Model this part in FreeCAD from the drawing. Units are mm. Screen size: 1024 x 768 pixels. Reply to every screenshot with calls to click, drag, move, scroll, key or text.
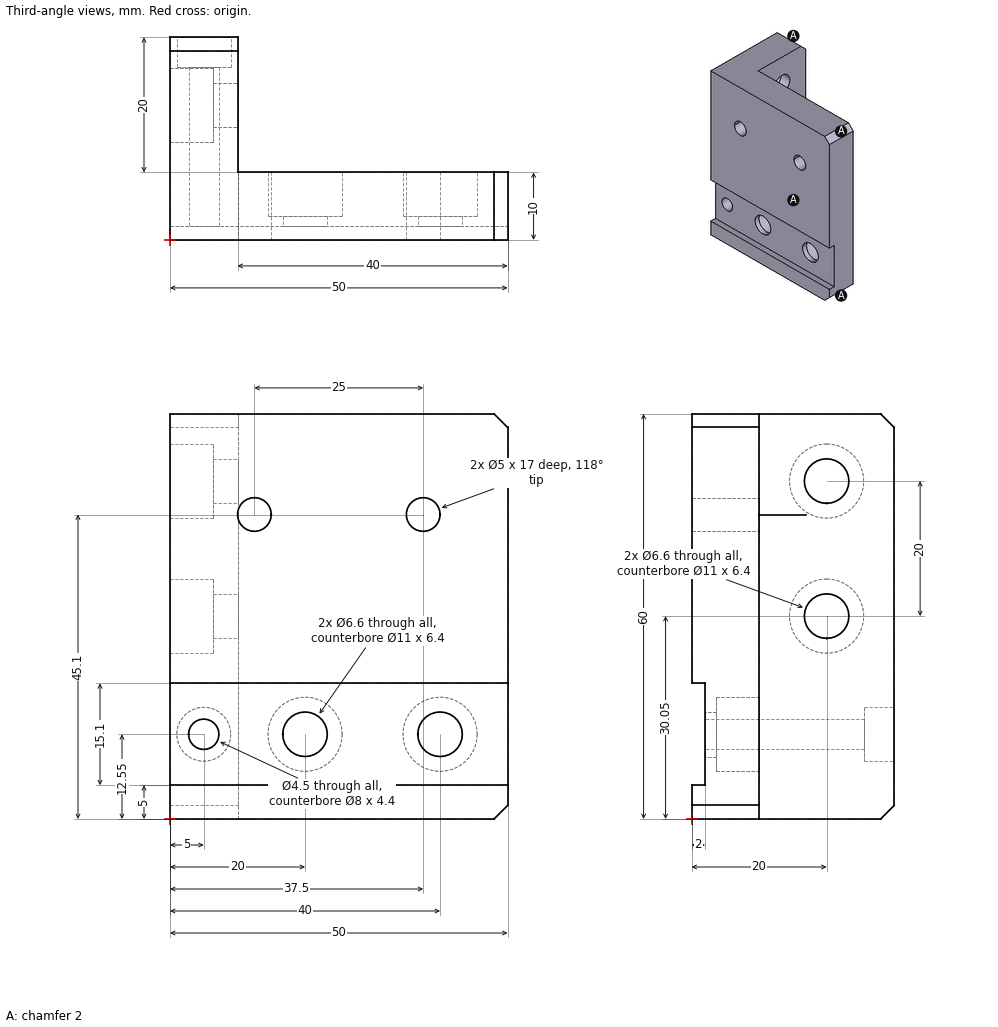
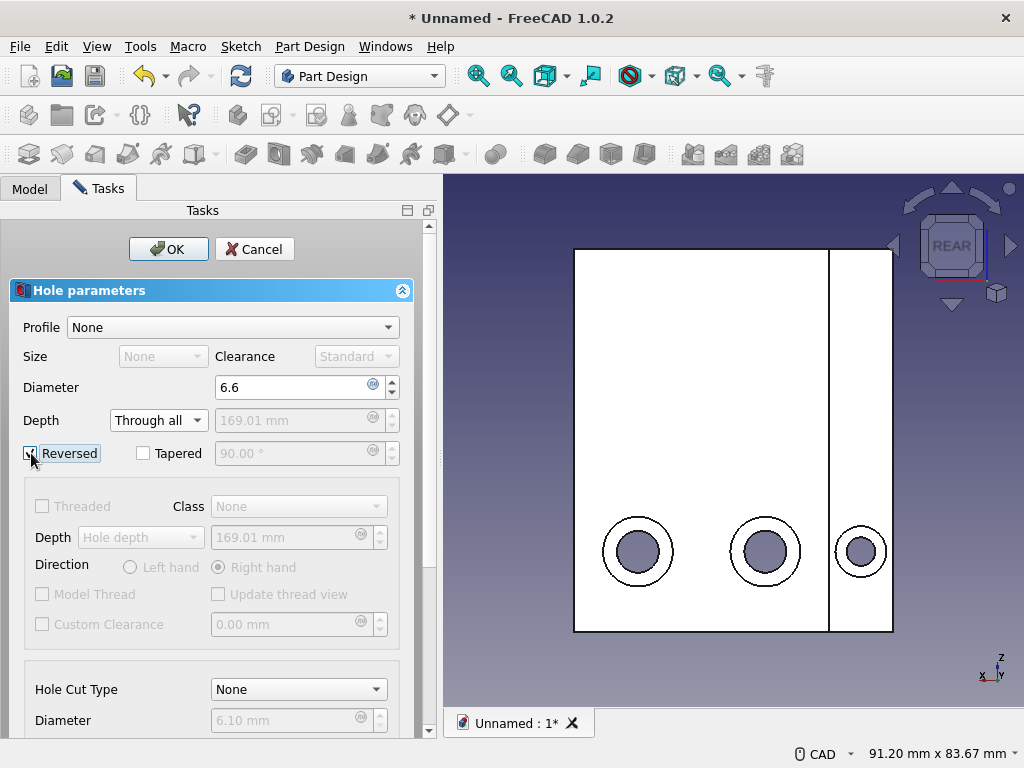
click(300, 690)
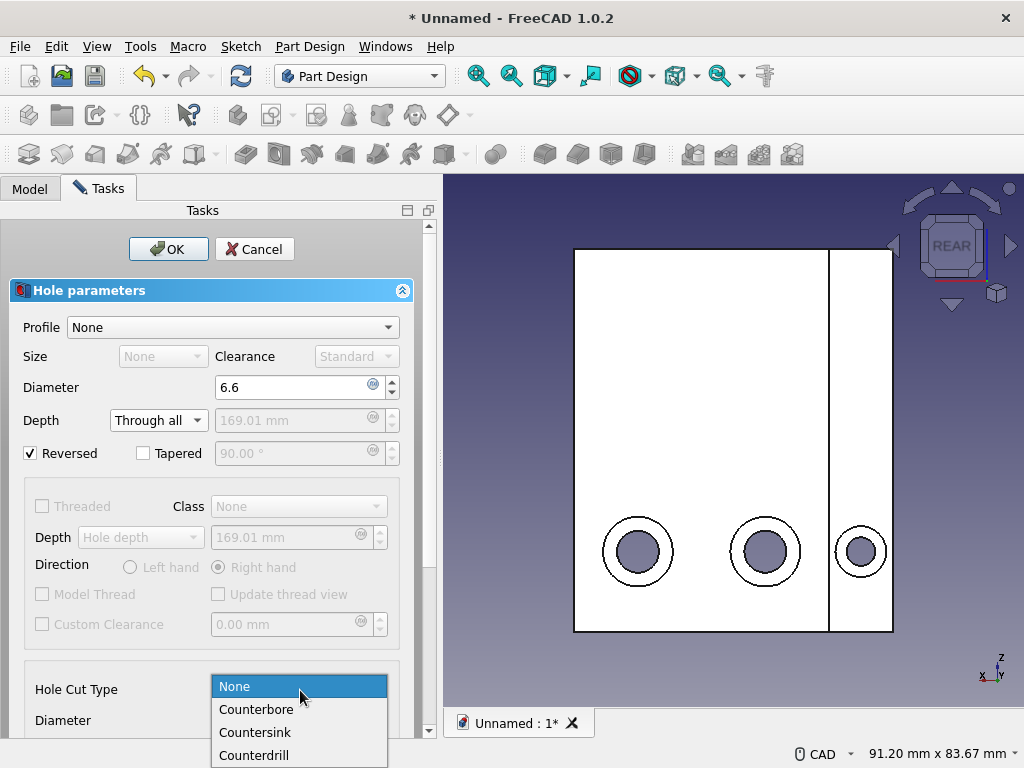
click(298, 710)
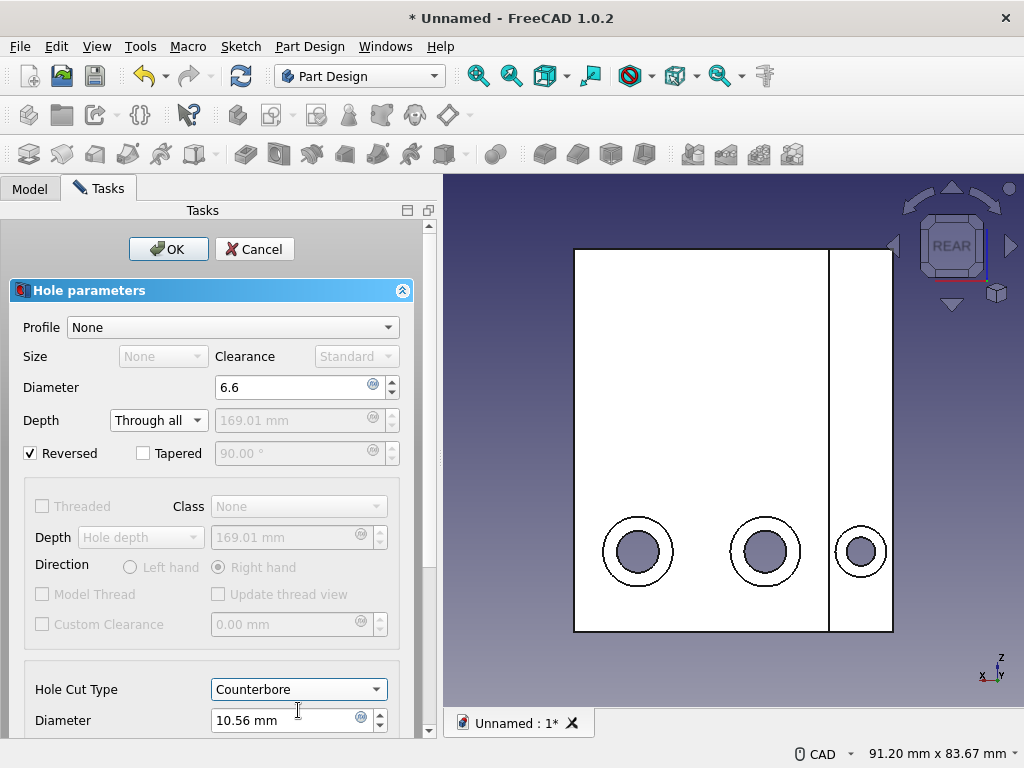
triple_click(292, 720)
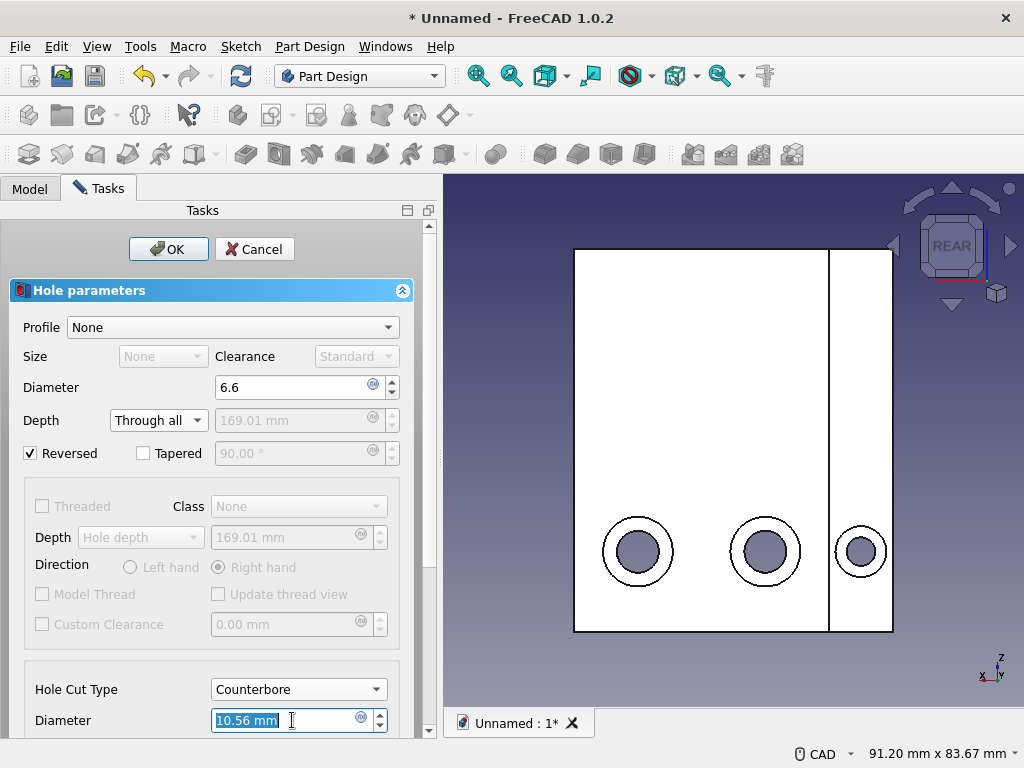
text(11)
key(Tab)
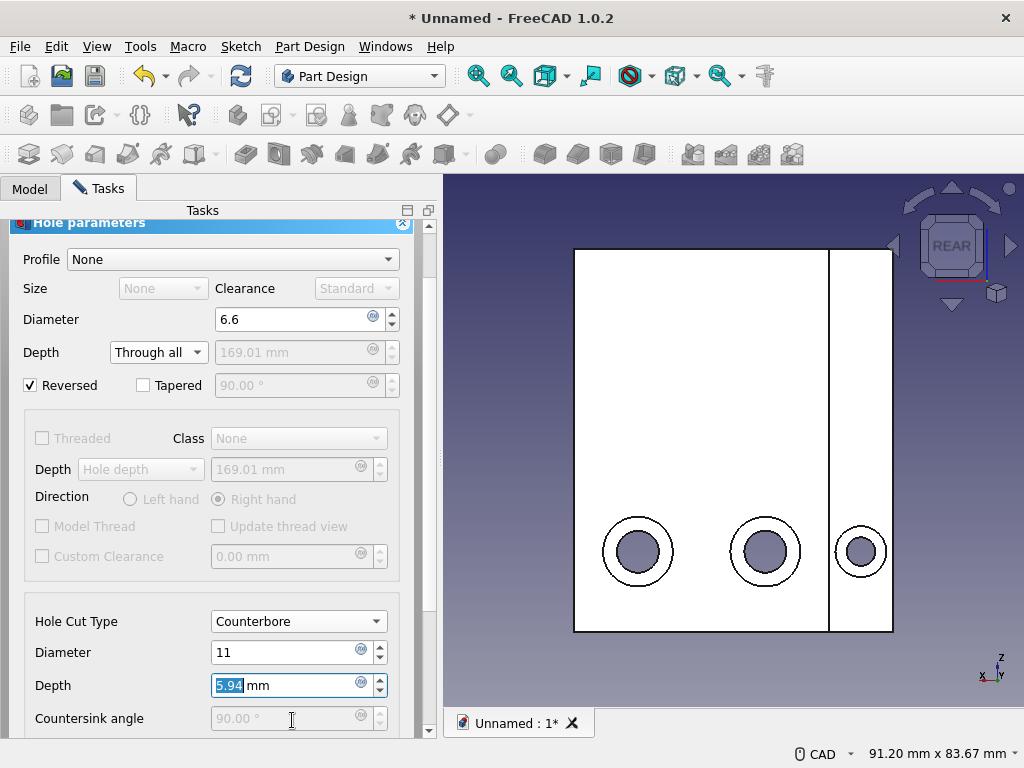
text(6.4)
key(Tab)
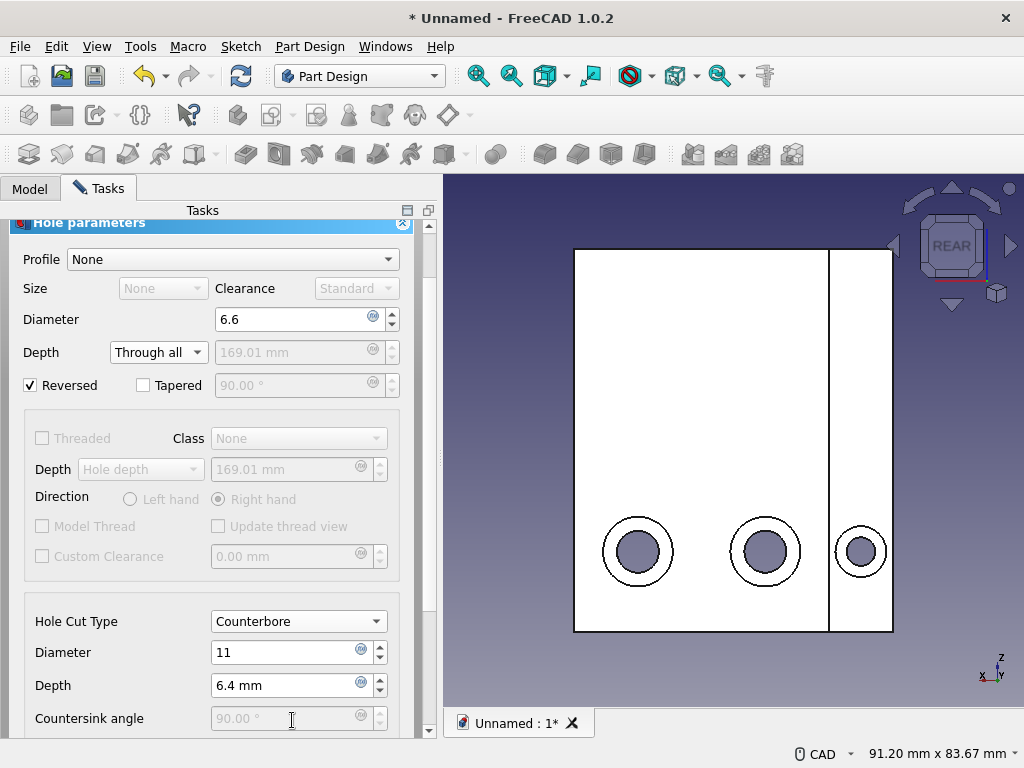
scroll(429, 479, up, 2)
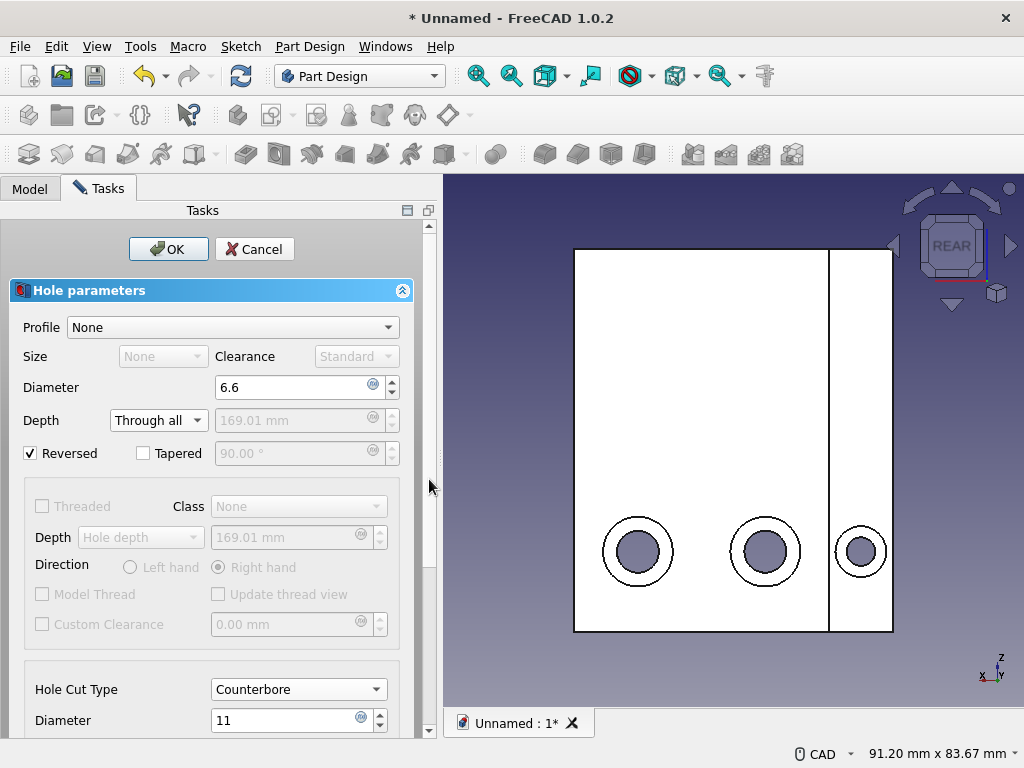
click(169, 249)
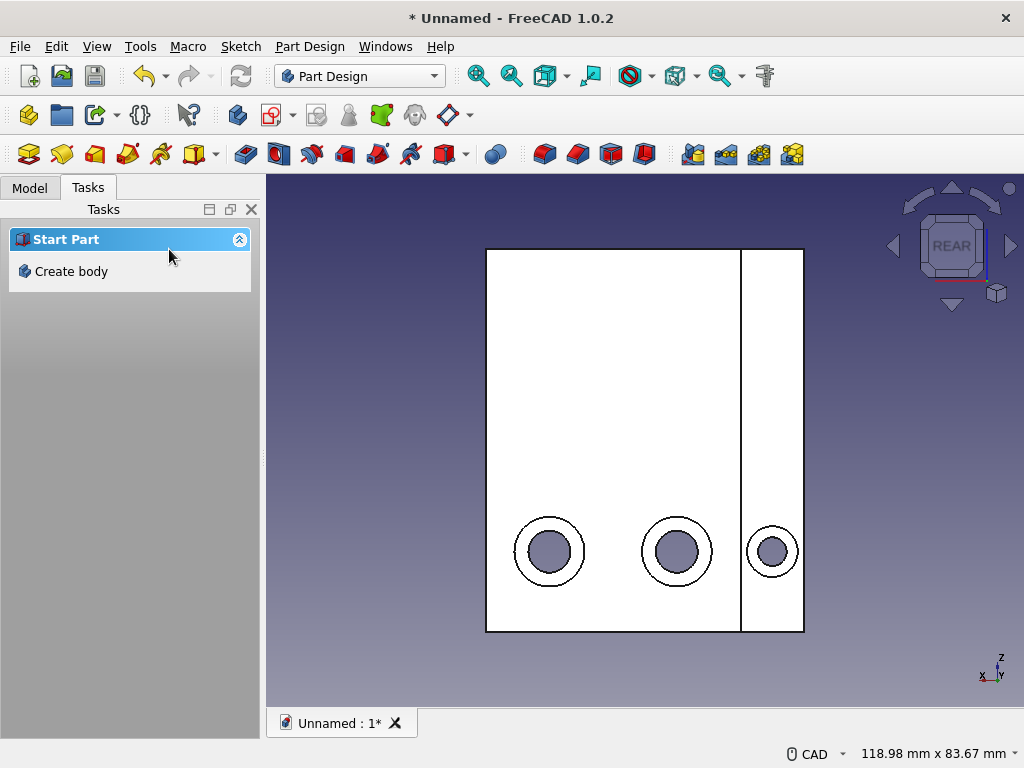
click(772, 248)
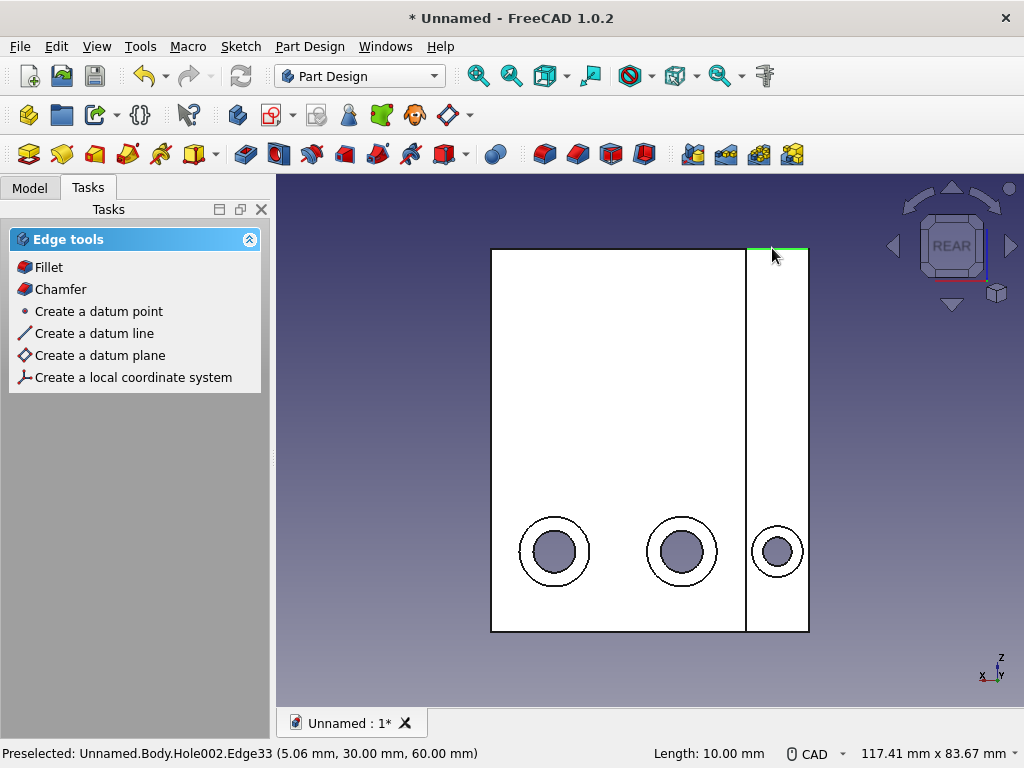
click(777, 631, ctrl)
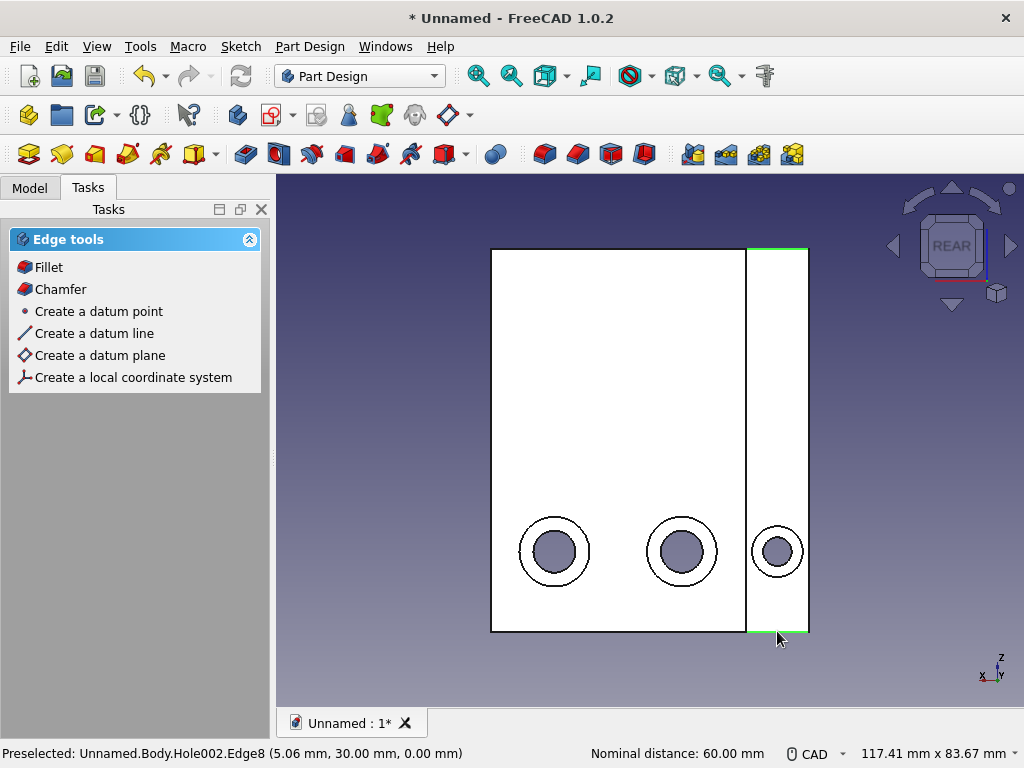
key(0)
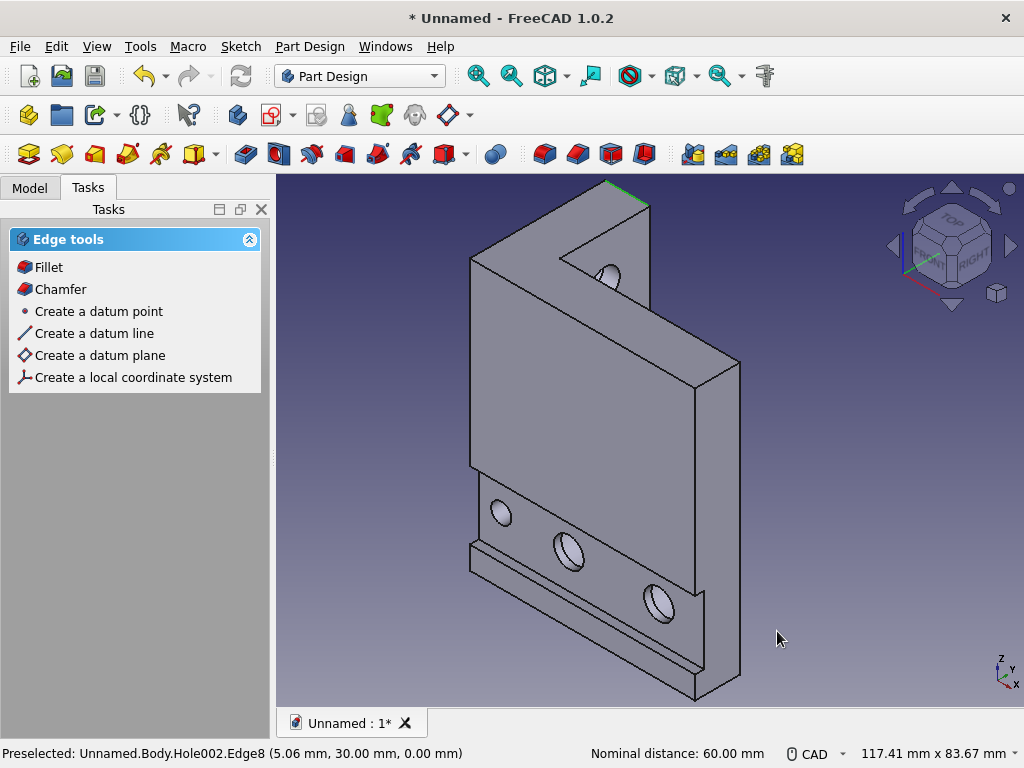
click(718, 374, ctrl)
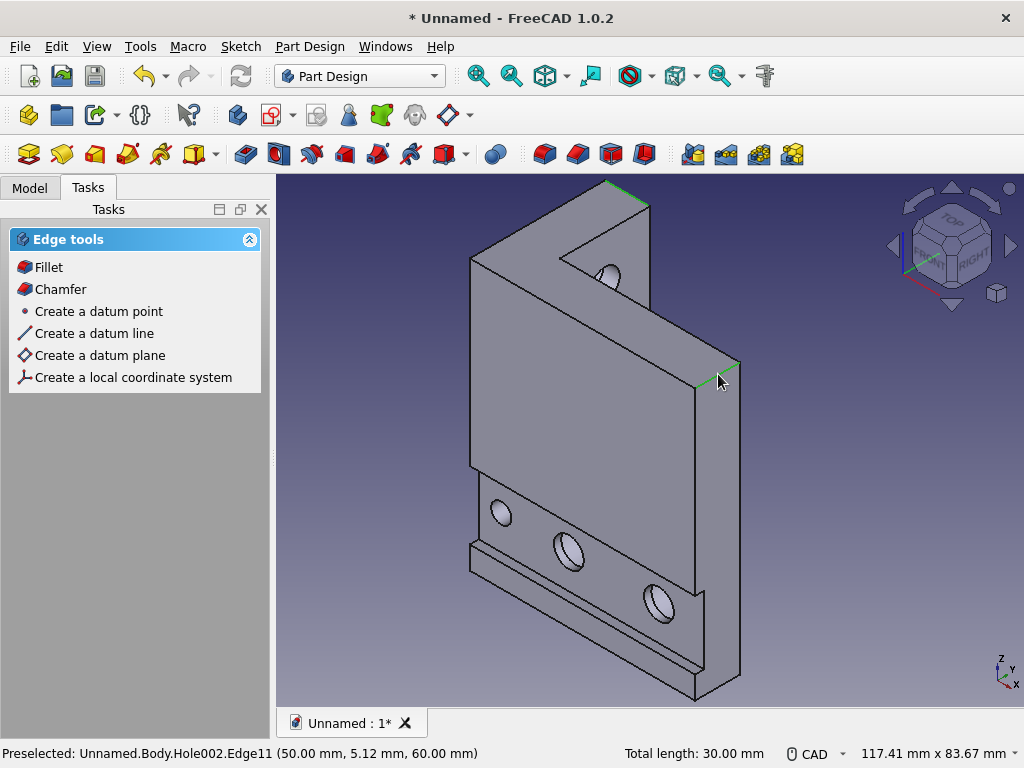
key(2)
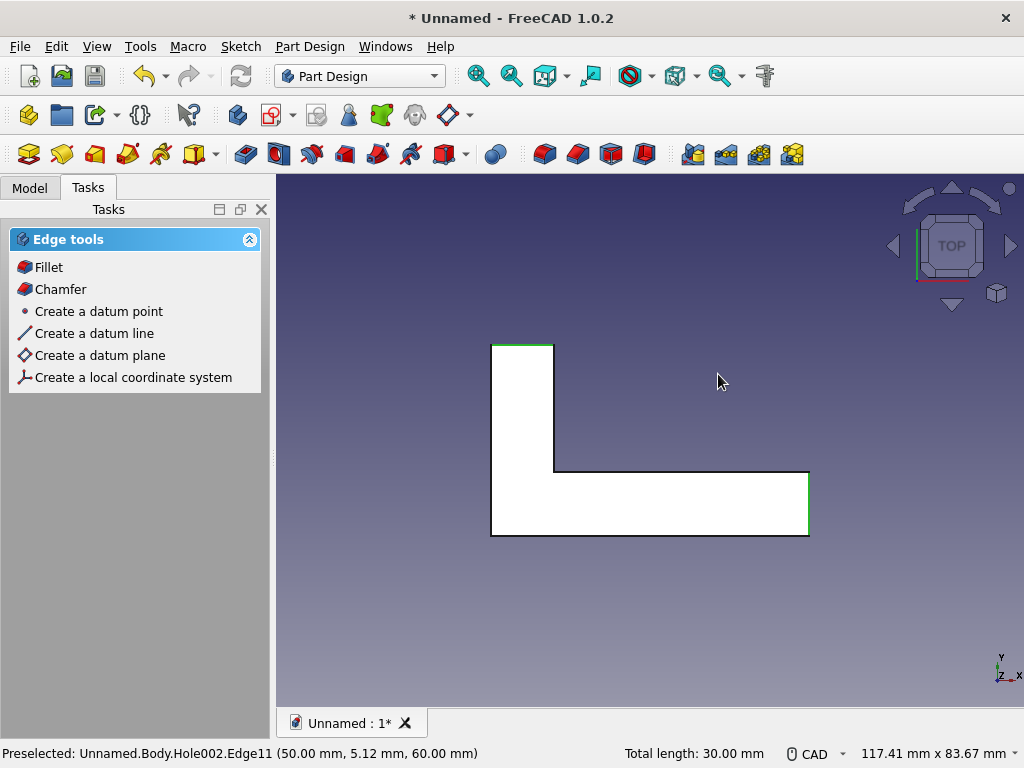
click(479, 76)